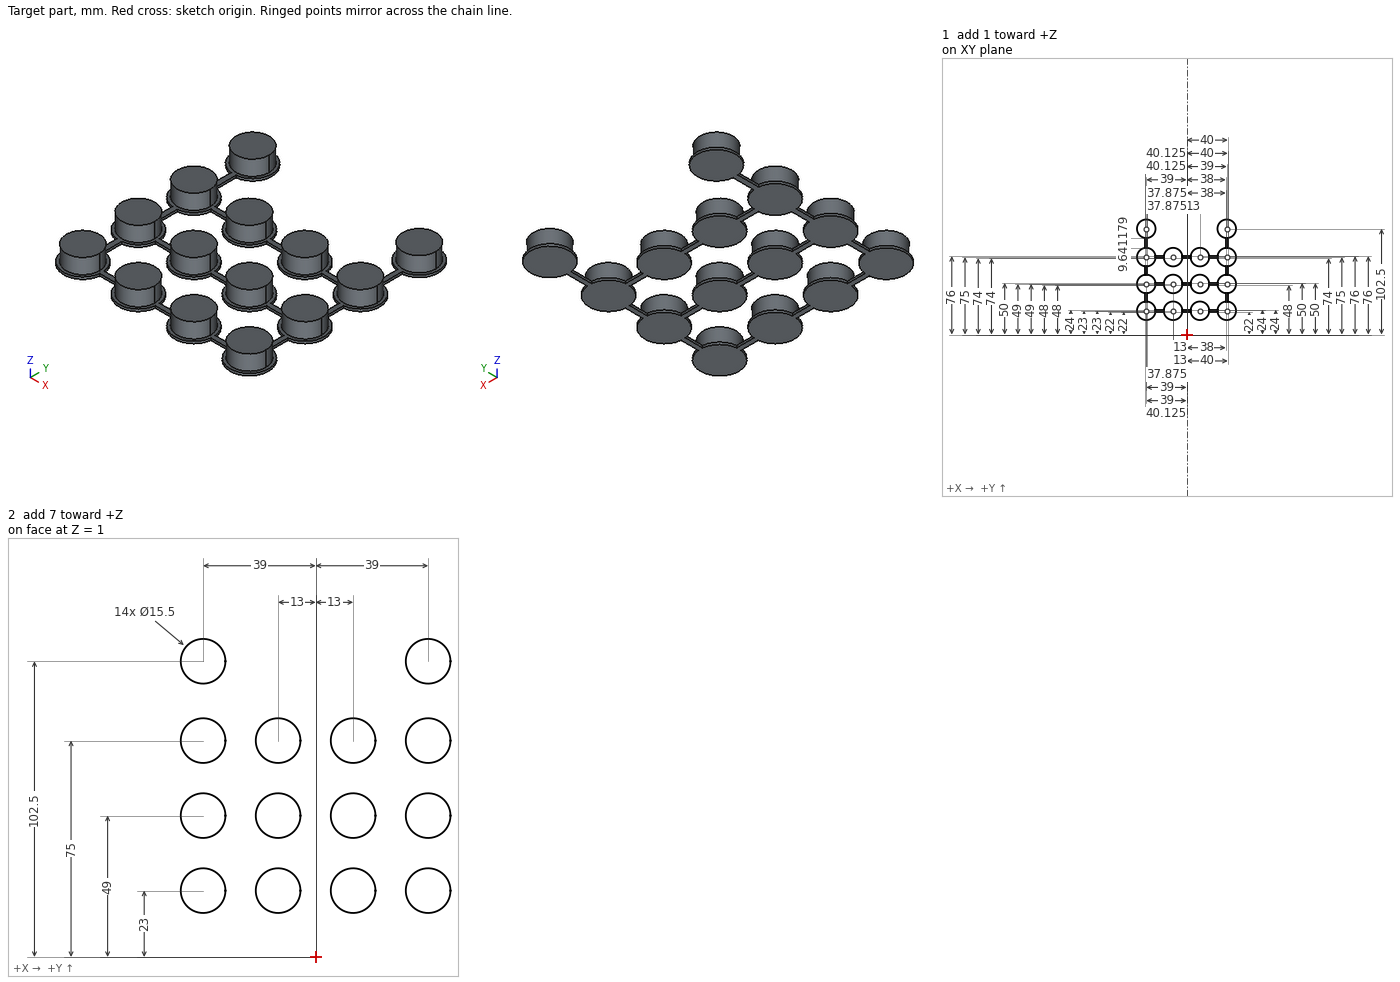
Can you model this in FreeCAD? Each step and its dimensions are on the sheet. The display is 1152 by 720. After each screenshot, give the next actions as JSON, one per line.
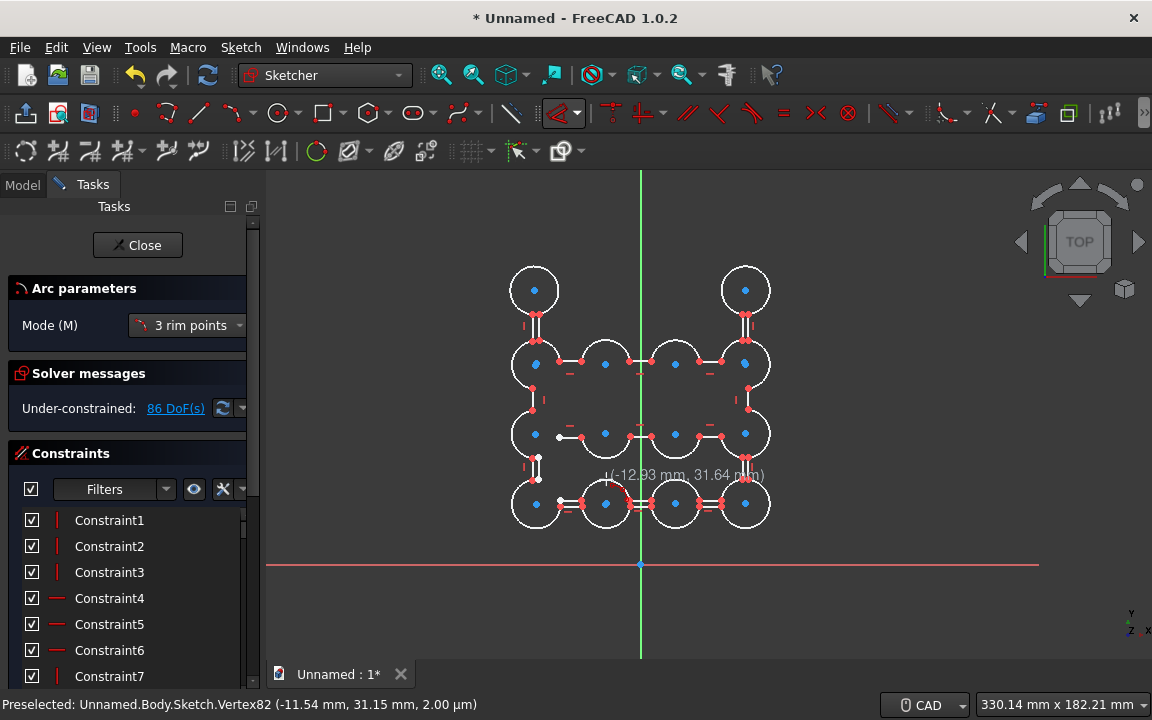
{"action": "scroll", "coordinate": [560, 500], "scroll_direction": "up", "scroll_amount": 6}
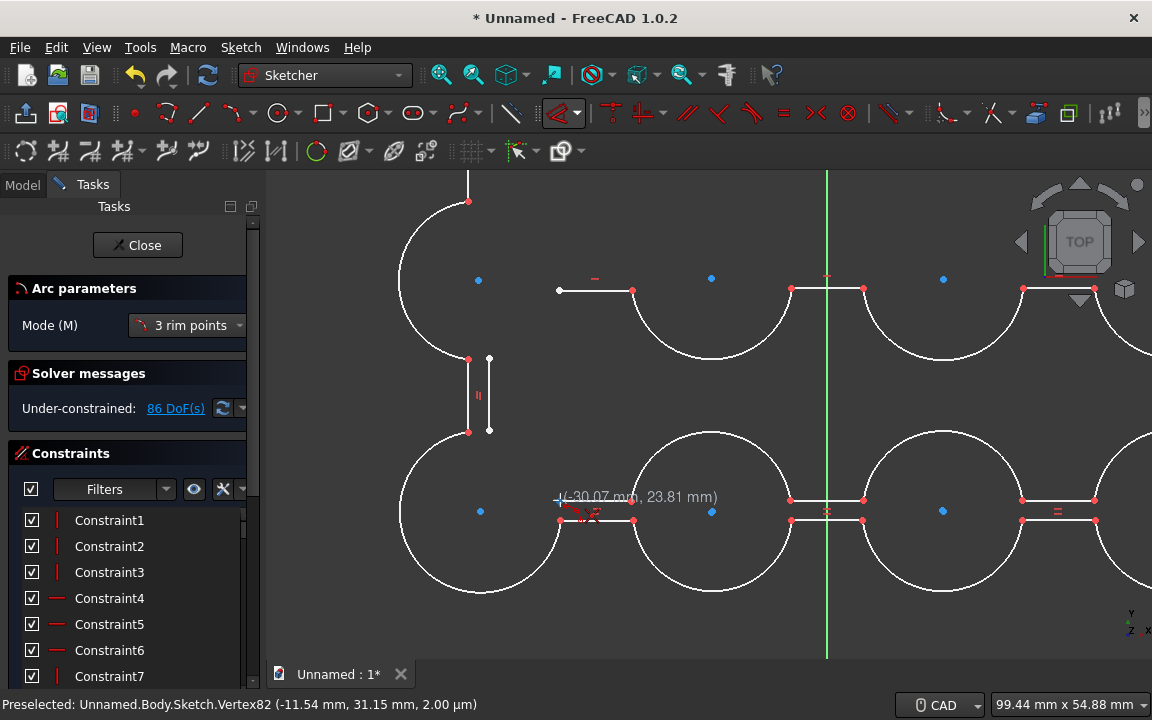
{"action": "left_click", "coordinate": [559, 501]}
{"action": "left_click", "coordinate": [489, 430]}
{"action": "left_click", "coordinate": [537, 453]}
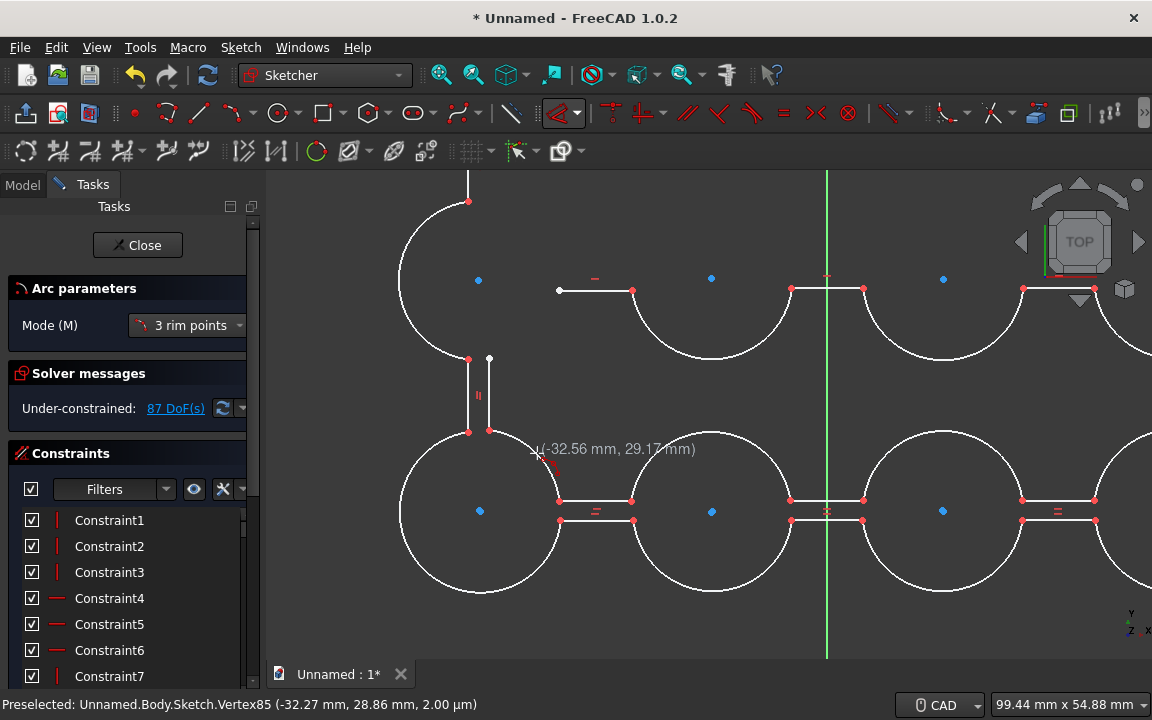
{"action": "left_click", "coordinate": [489, 358]}
{"action": "left_click", "coordinate": [559, 291]}
{"action": "left_click", "coordinate": [537, 334]}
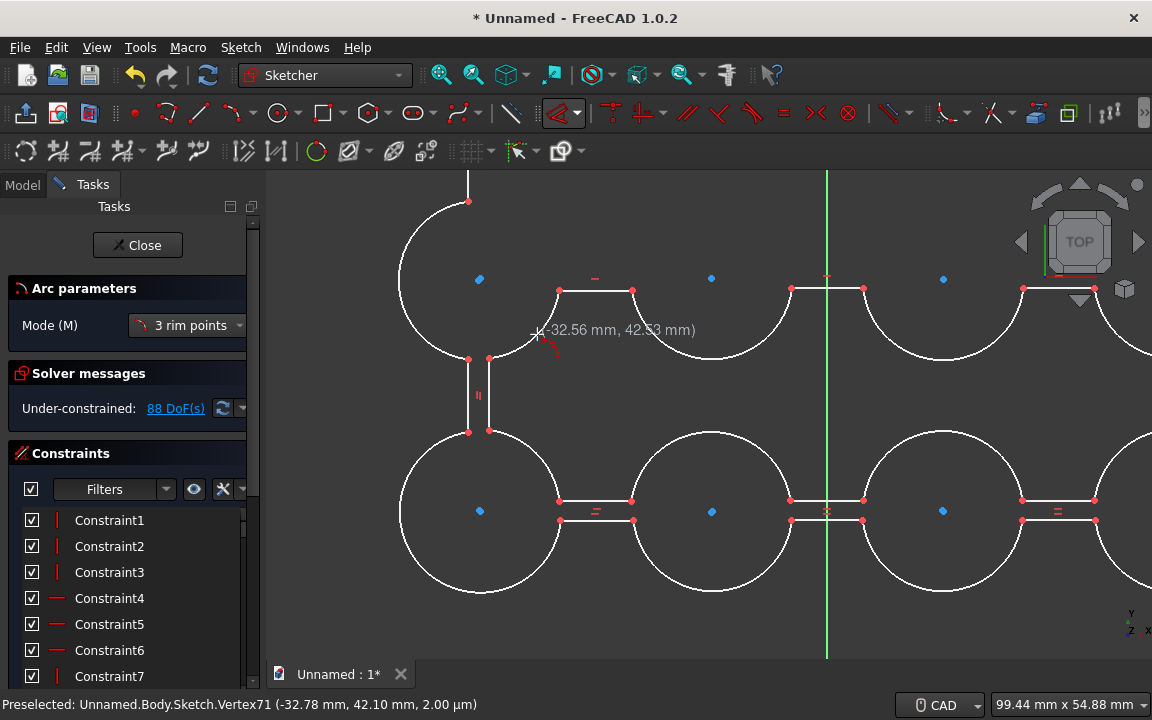
{"action": "left_click", "coordinate": [200, 114]}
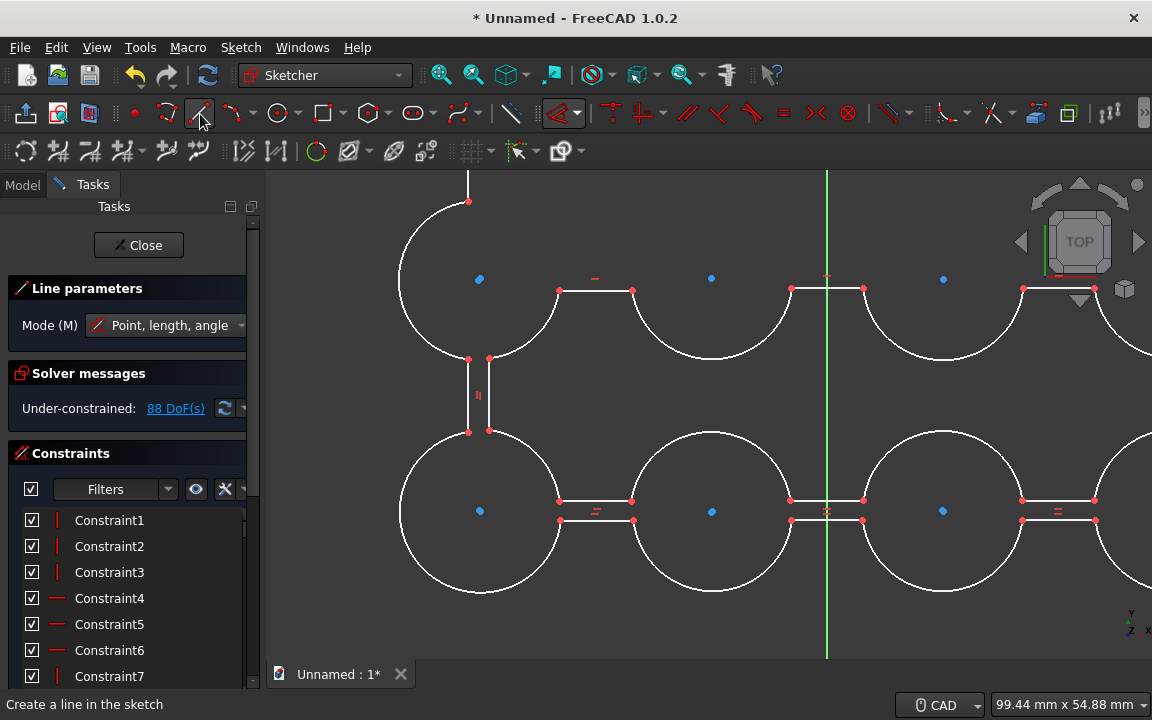
{"action": "scroll", "coordinate": [560, 500], "scroll_direction": "down", "scroll_amount": 6}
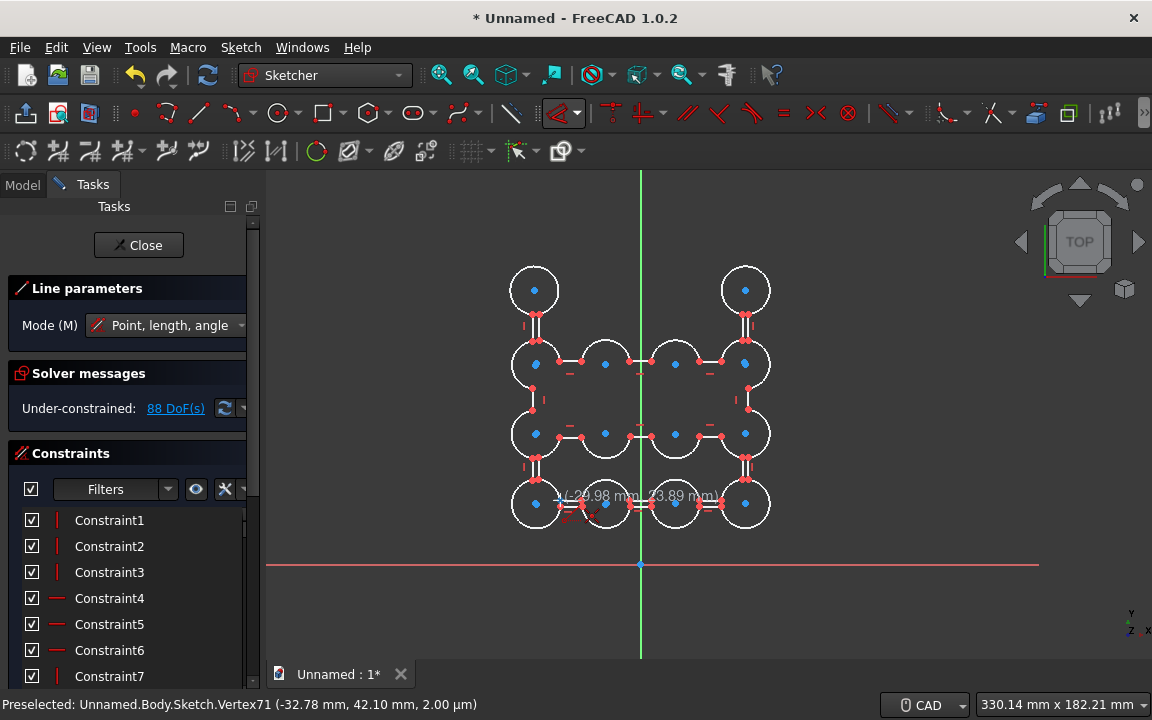
{"action": "scroll", "coordinate": [560, 366], "scroll_direction": "up", "scroll_amount": 6}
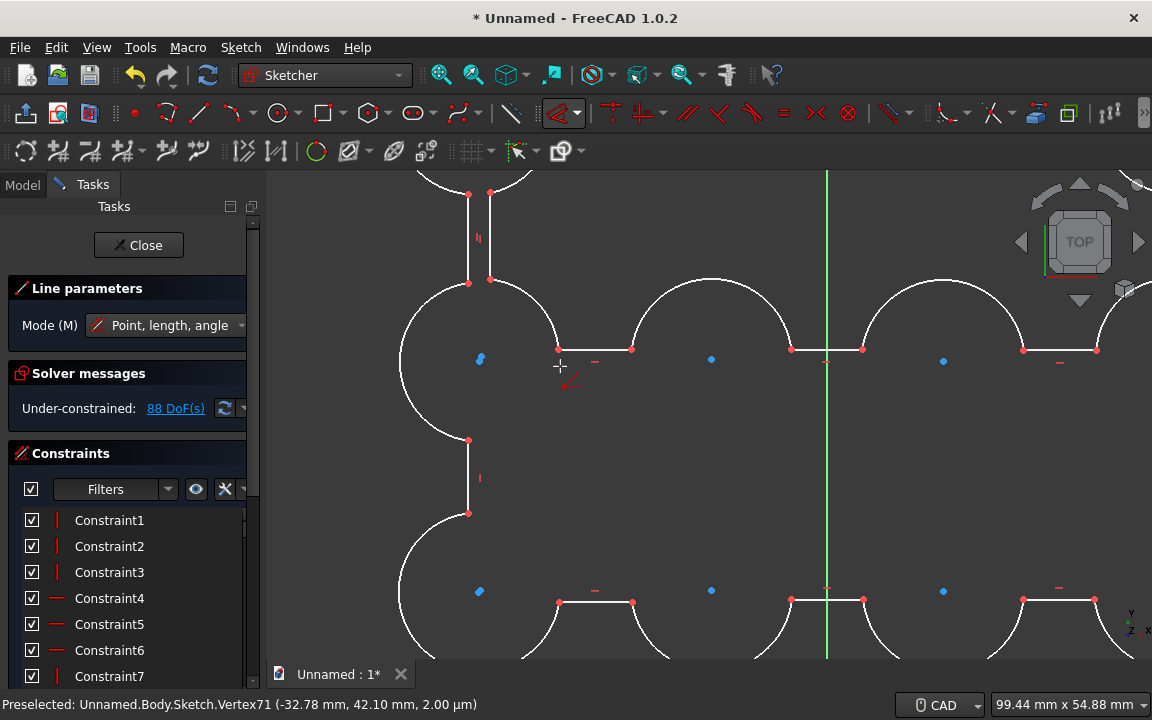
{"action": "left_click", "coordinate": [559, 366]}
{"action": "left_click", "coordinate": [632, 366]}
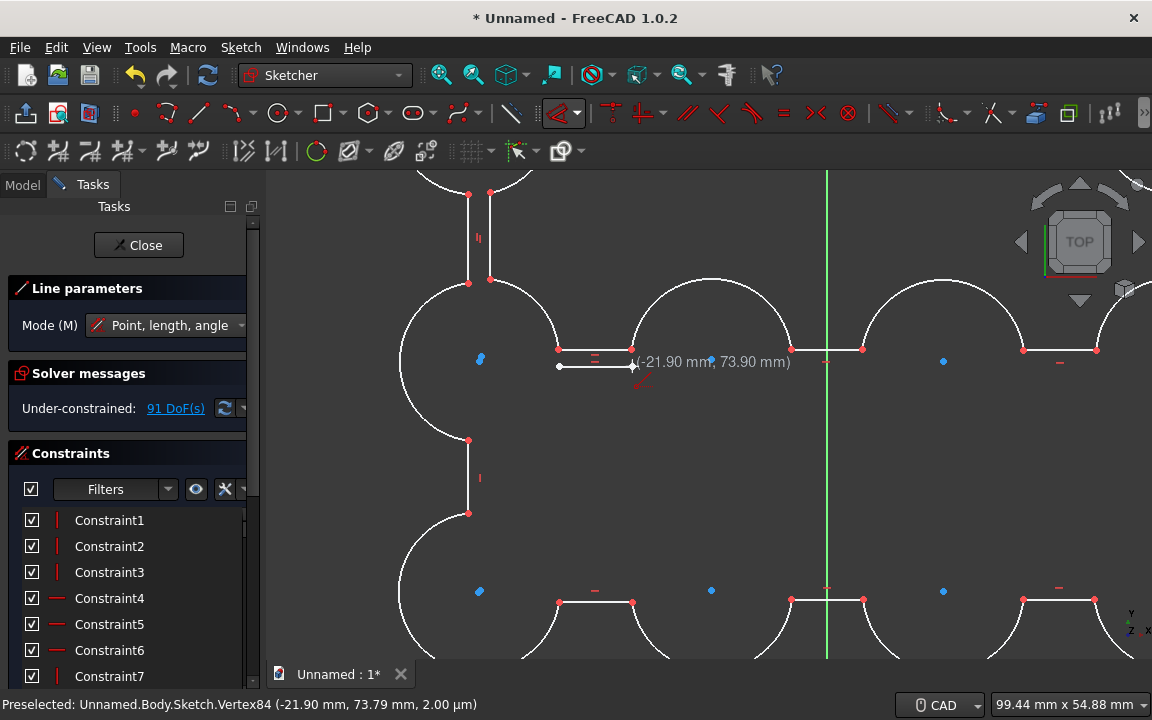
{"action": "left_click", "coordinate": [791, 366]}
{"action": "left_click", "coordinate": [863, 366]}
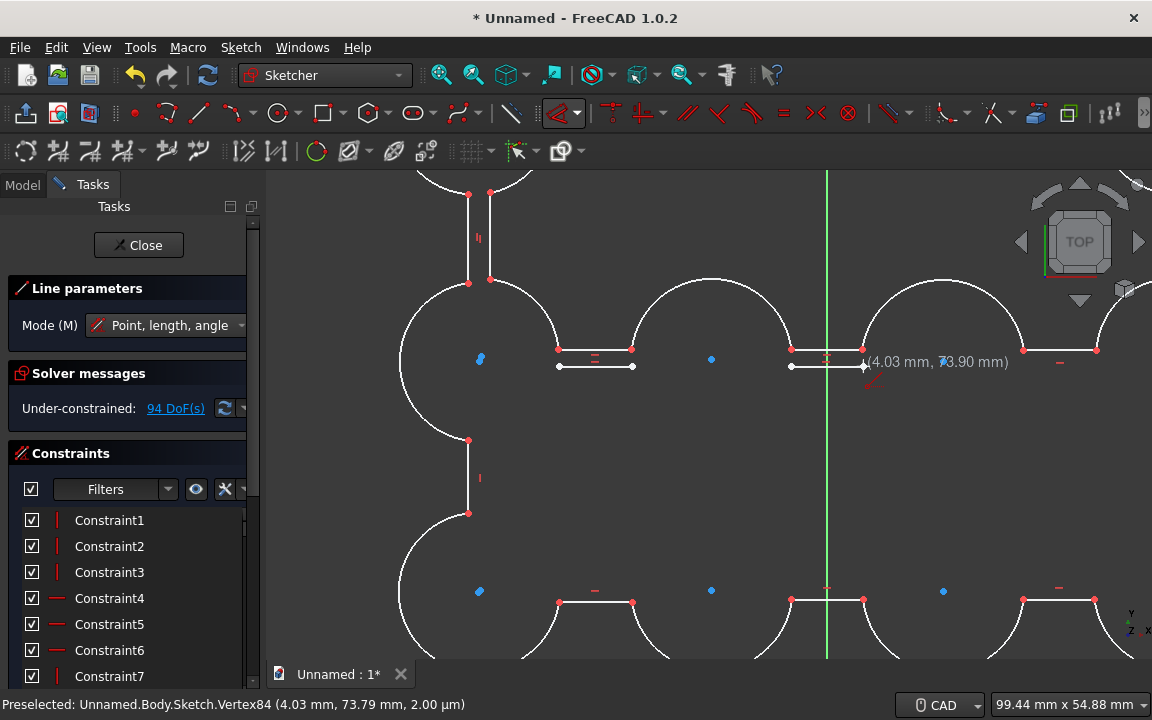
{"action": "scroll", "coordinate": [560, 365], "scroll_direction": "down", "scroll_amount": 6}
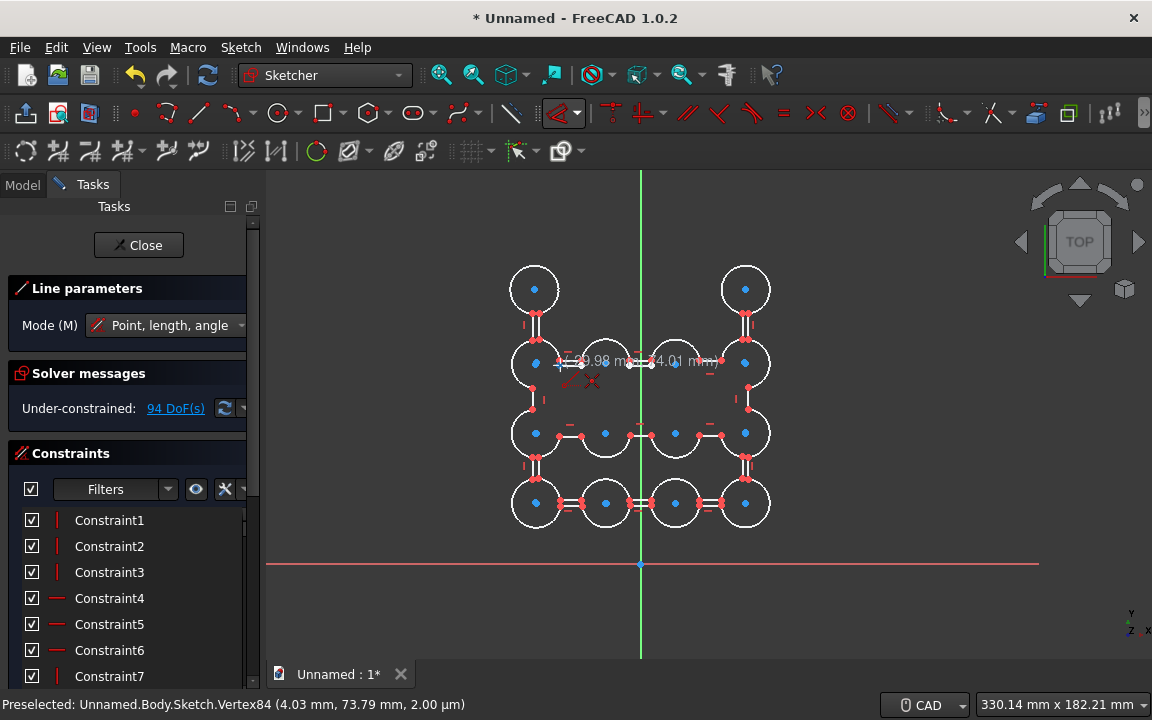
{"action": "scroll", "coordinate": [700, 366], "scroll_direction": "up", "scroll_amount": 6}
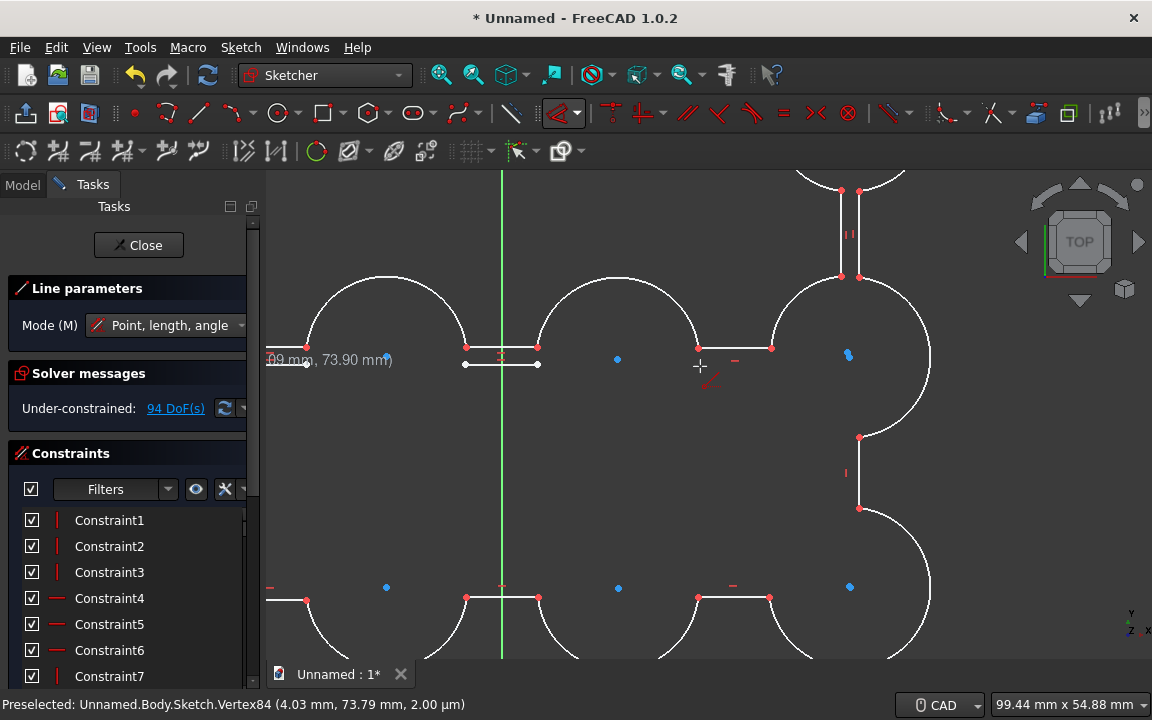
{"action": "left_click", "coordinate": [697, 364]}
{"action": "left_click", "coordinate": [770, 364]}